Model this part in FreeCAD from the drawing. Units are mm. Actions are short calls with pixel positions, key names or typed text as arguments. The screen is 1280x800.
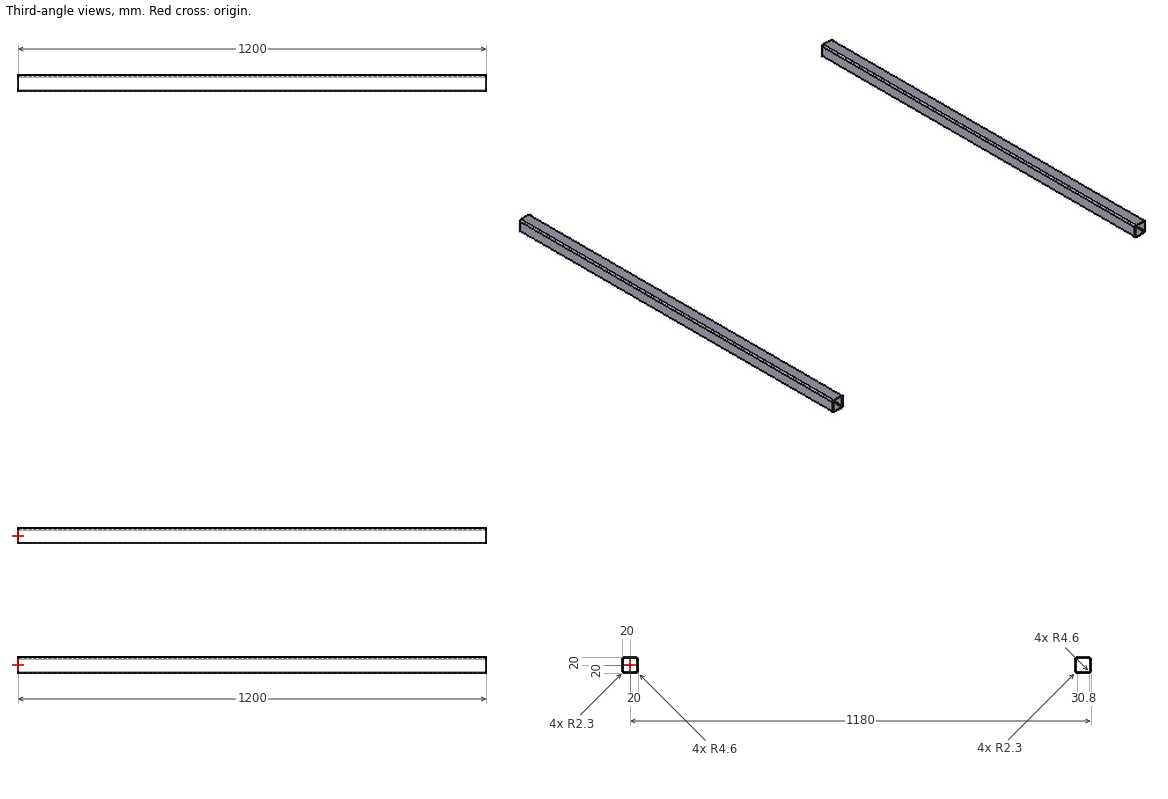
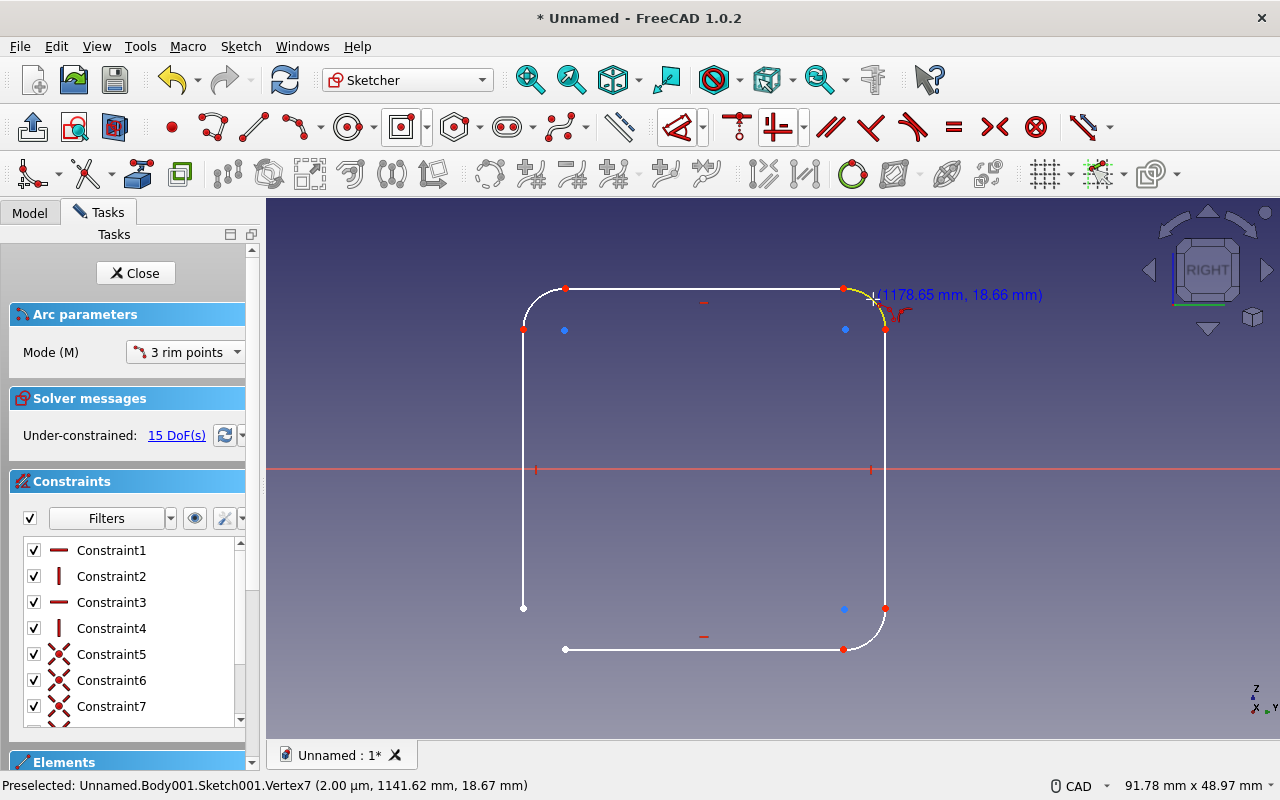
click(523, 609)
click(565, 650)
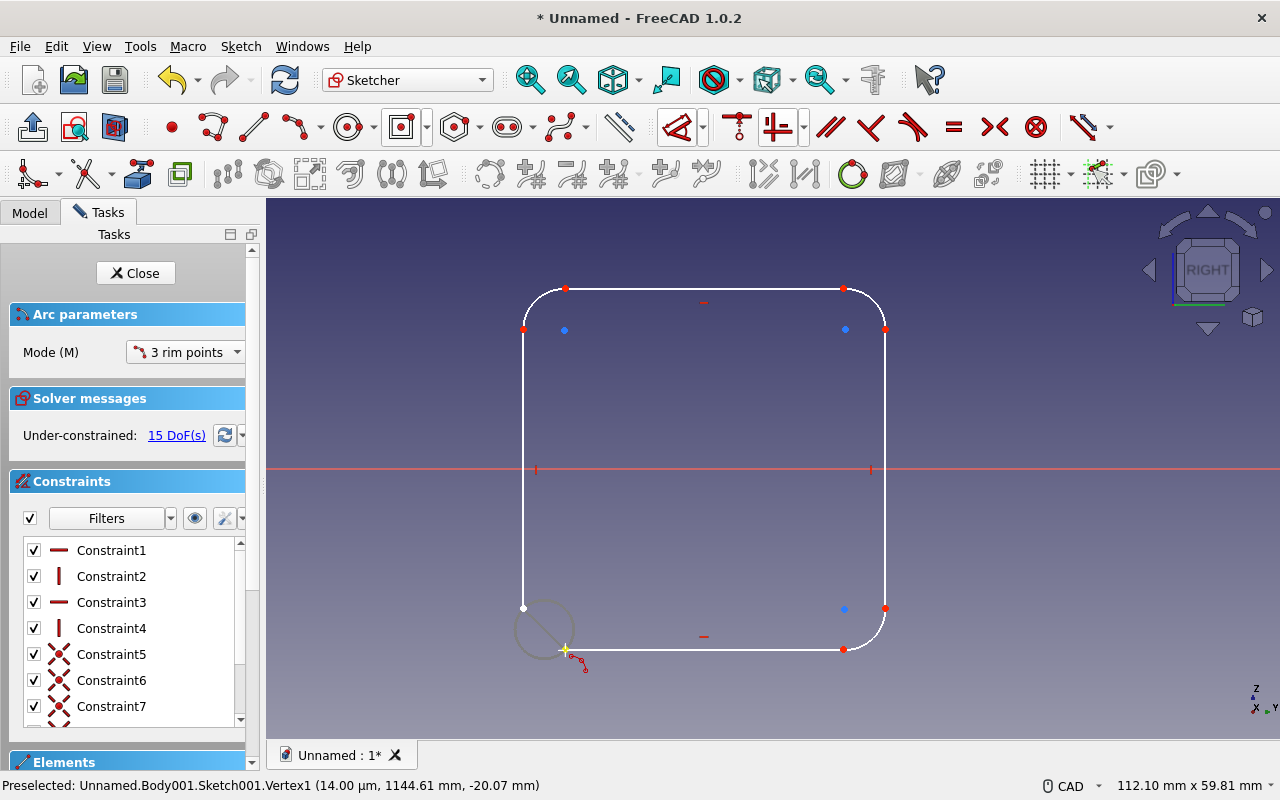
scroll(536, 637, up, 2)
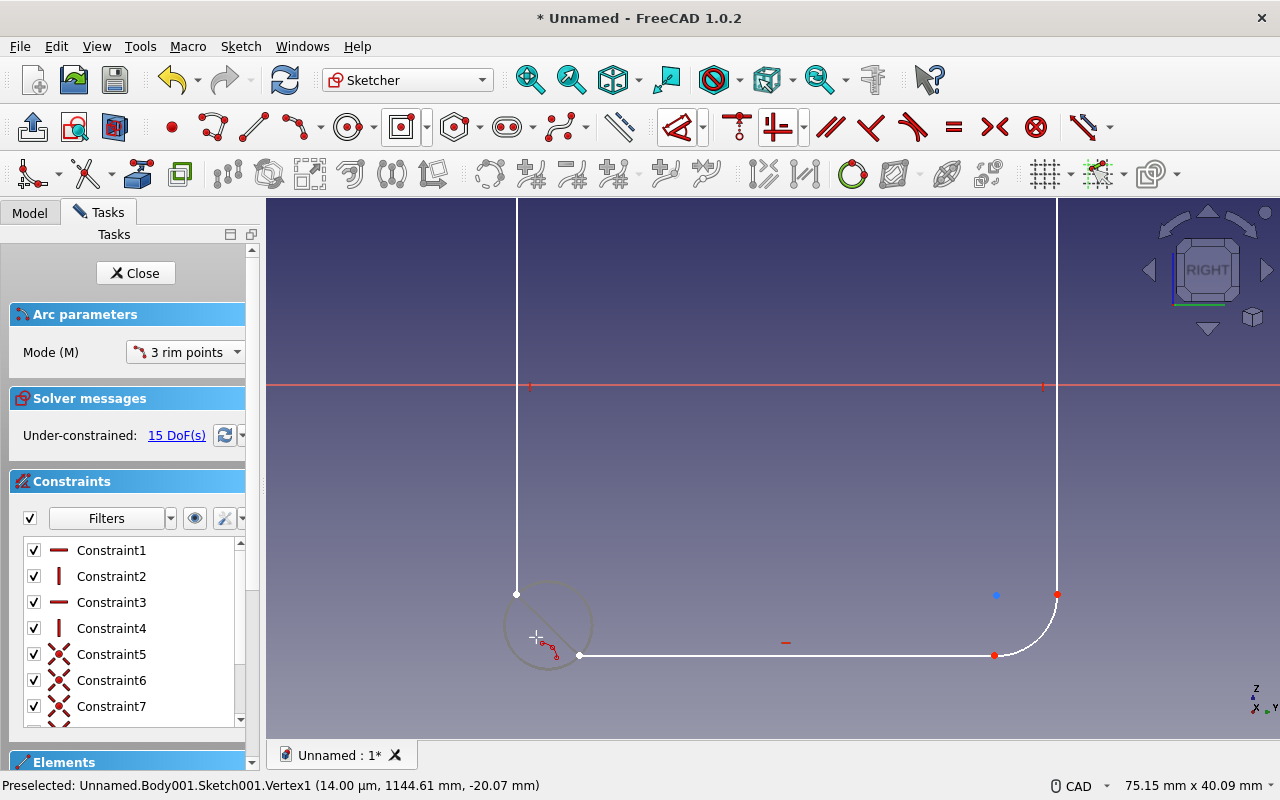
click(536, 637)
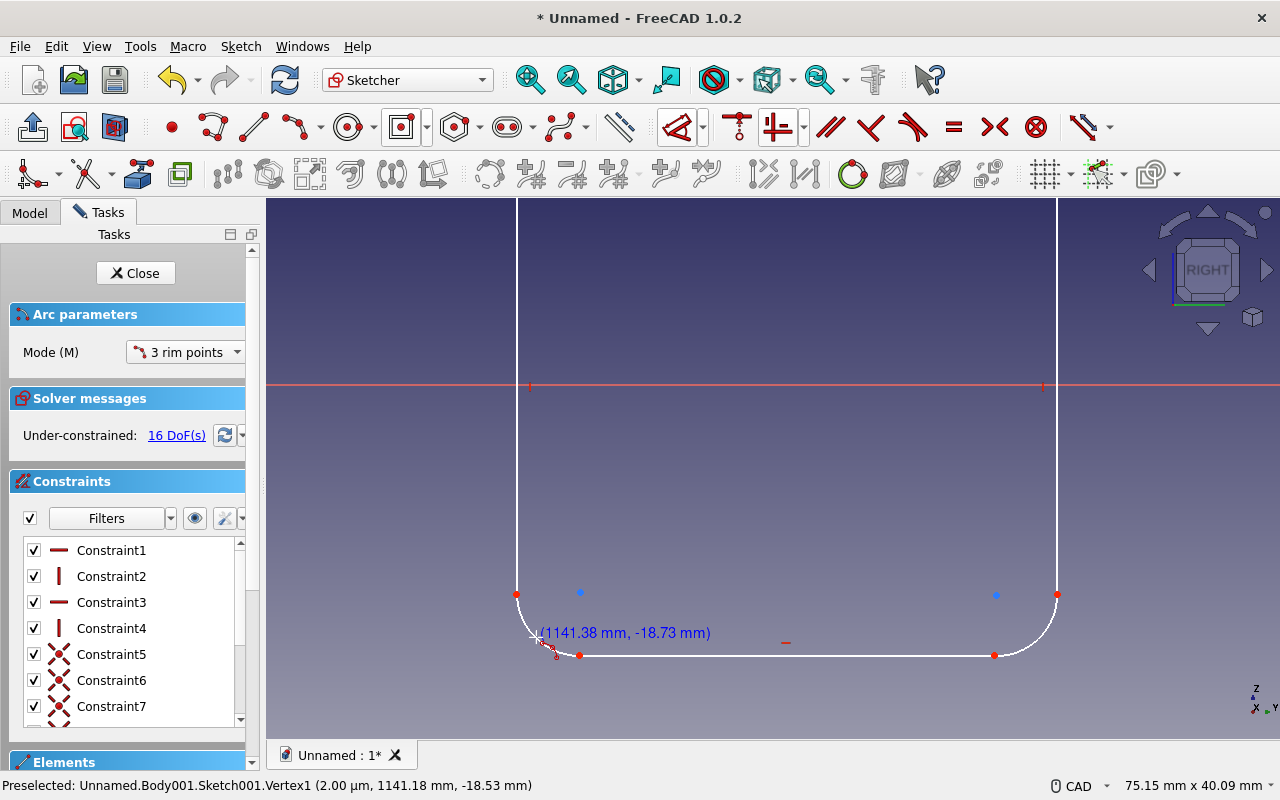
key(g)
key(l)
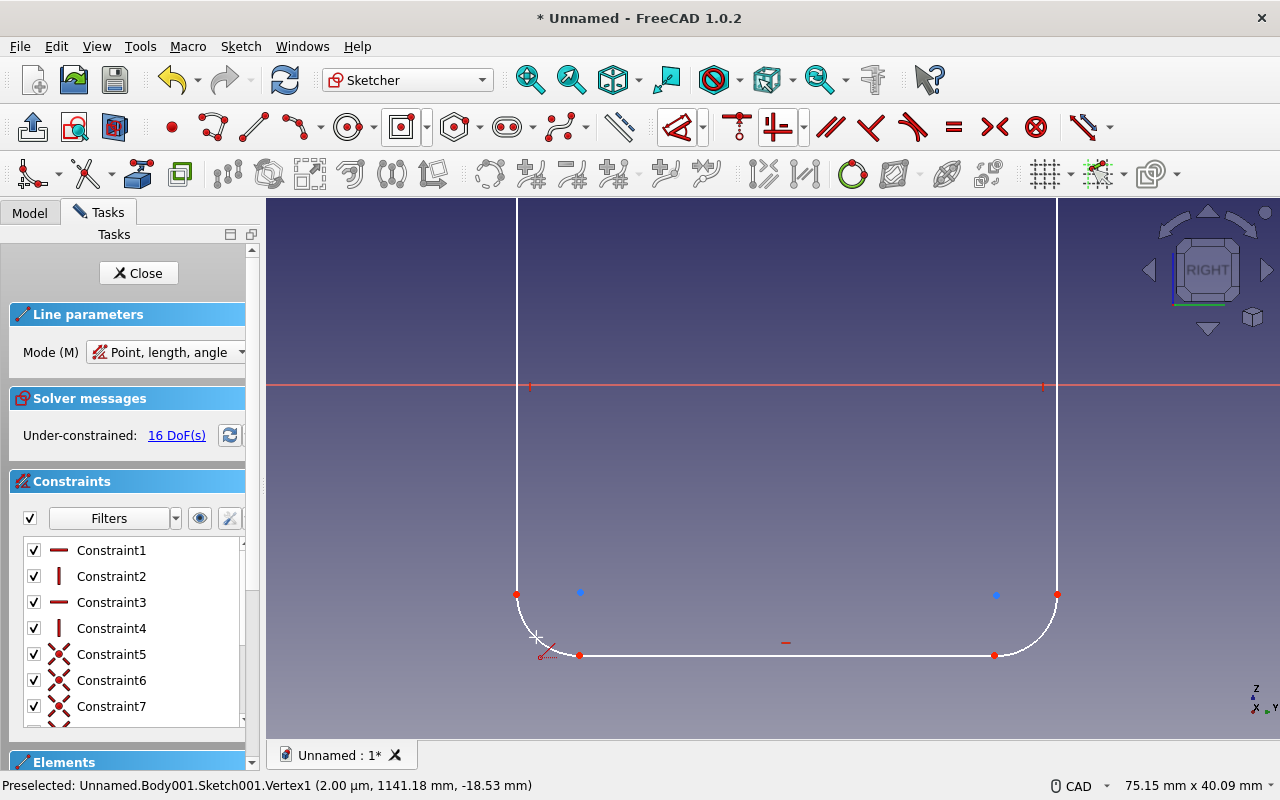
click(995, 624)
click(579, 624)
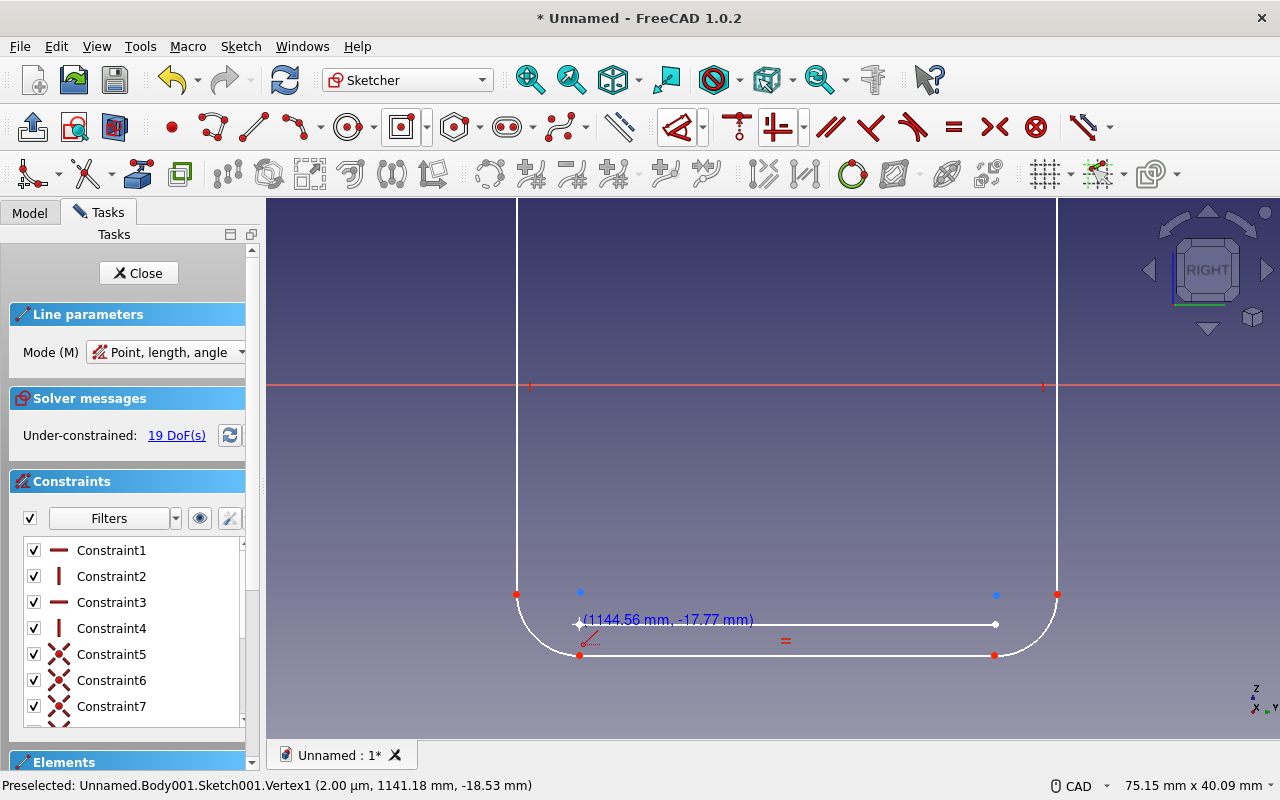
click(548, 593)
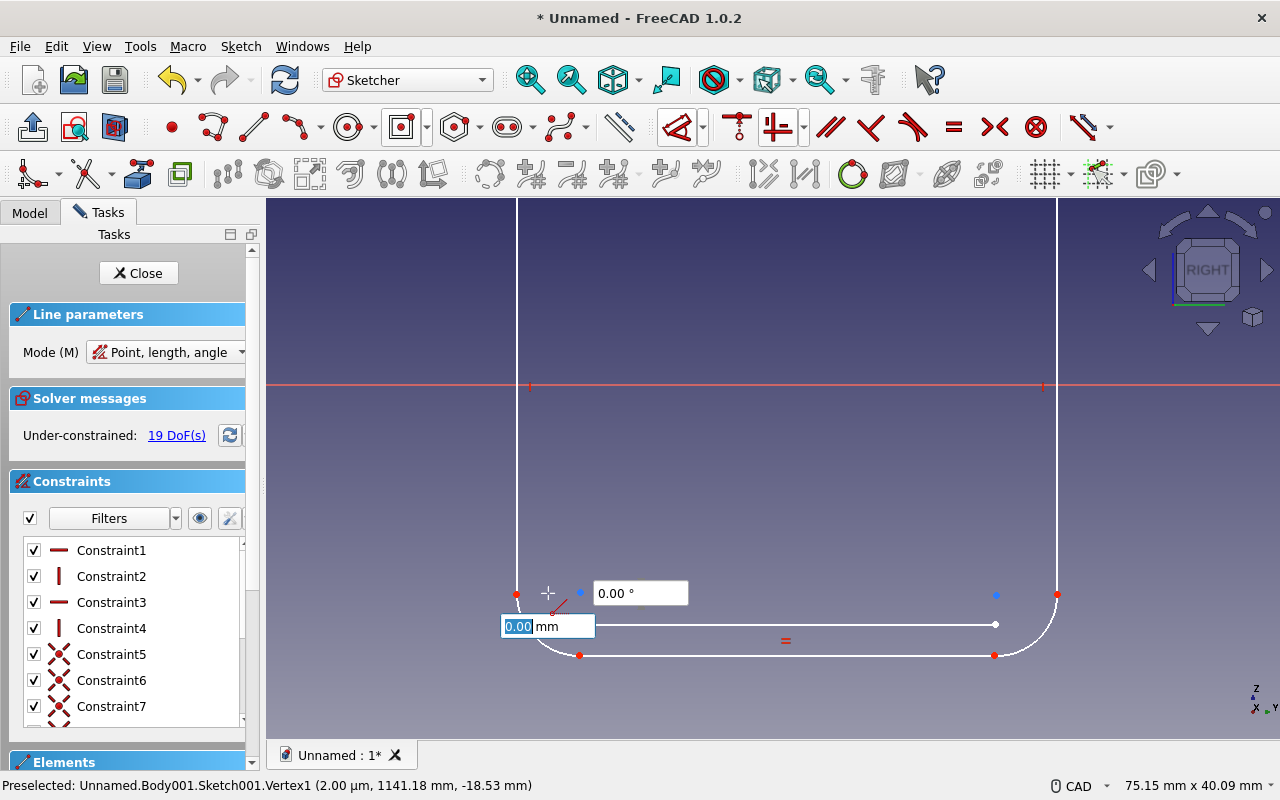
scroll(536, 638, down, 2)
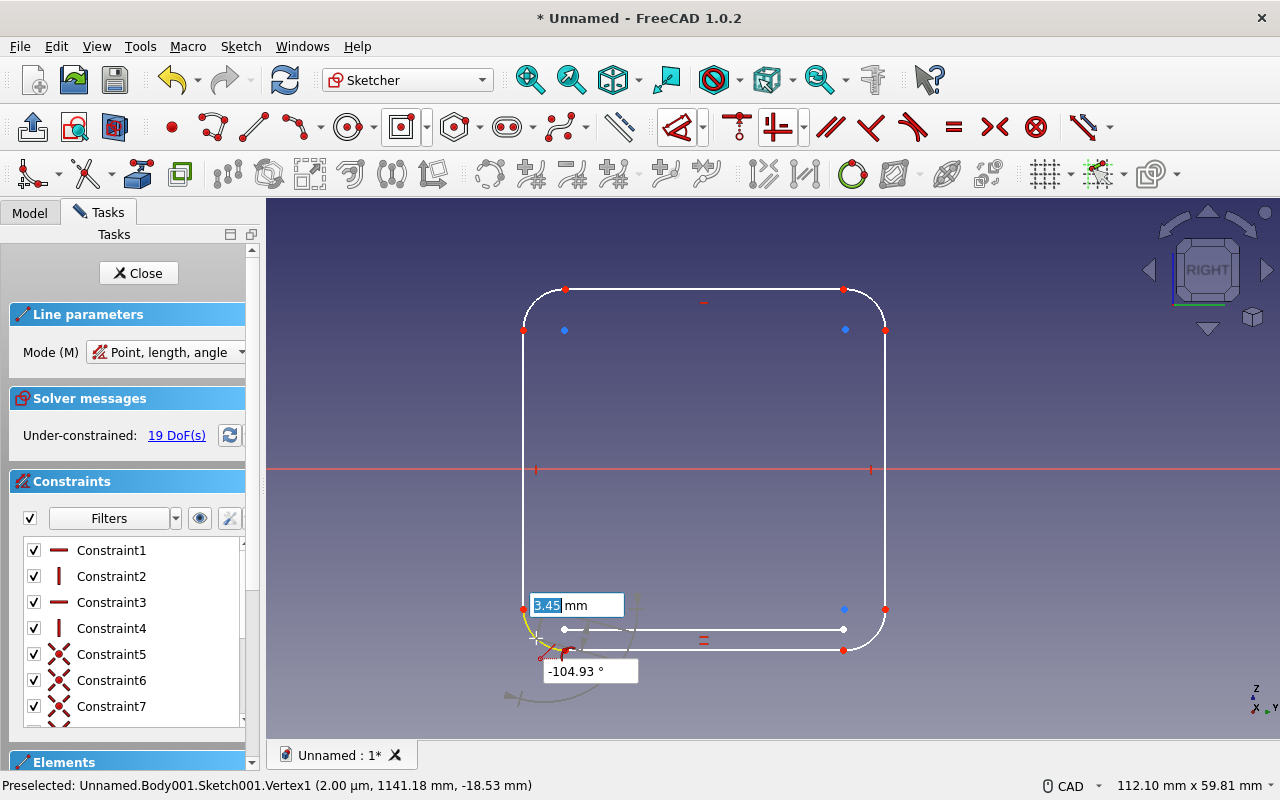
click(544, 330)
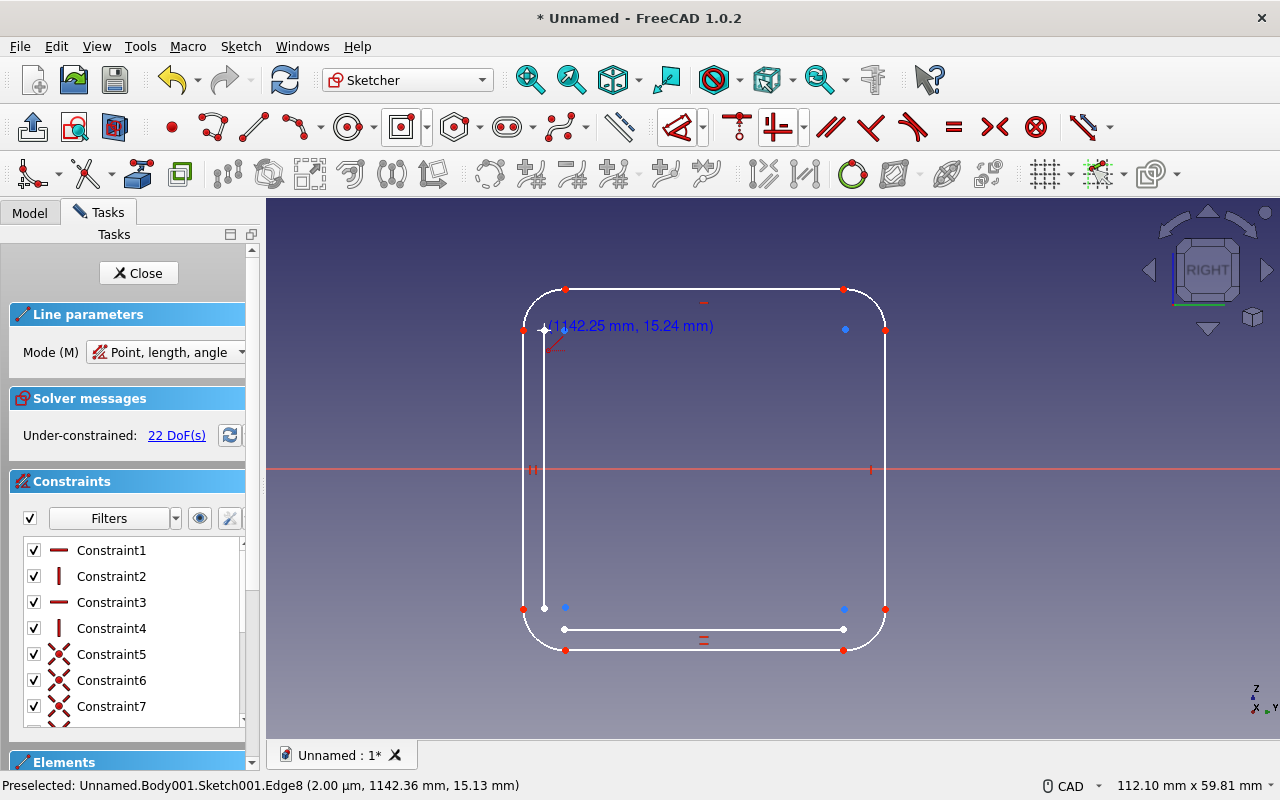
click(565, 309)
click(844, 309)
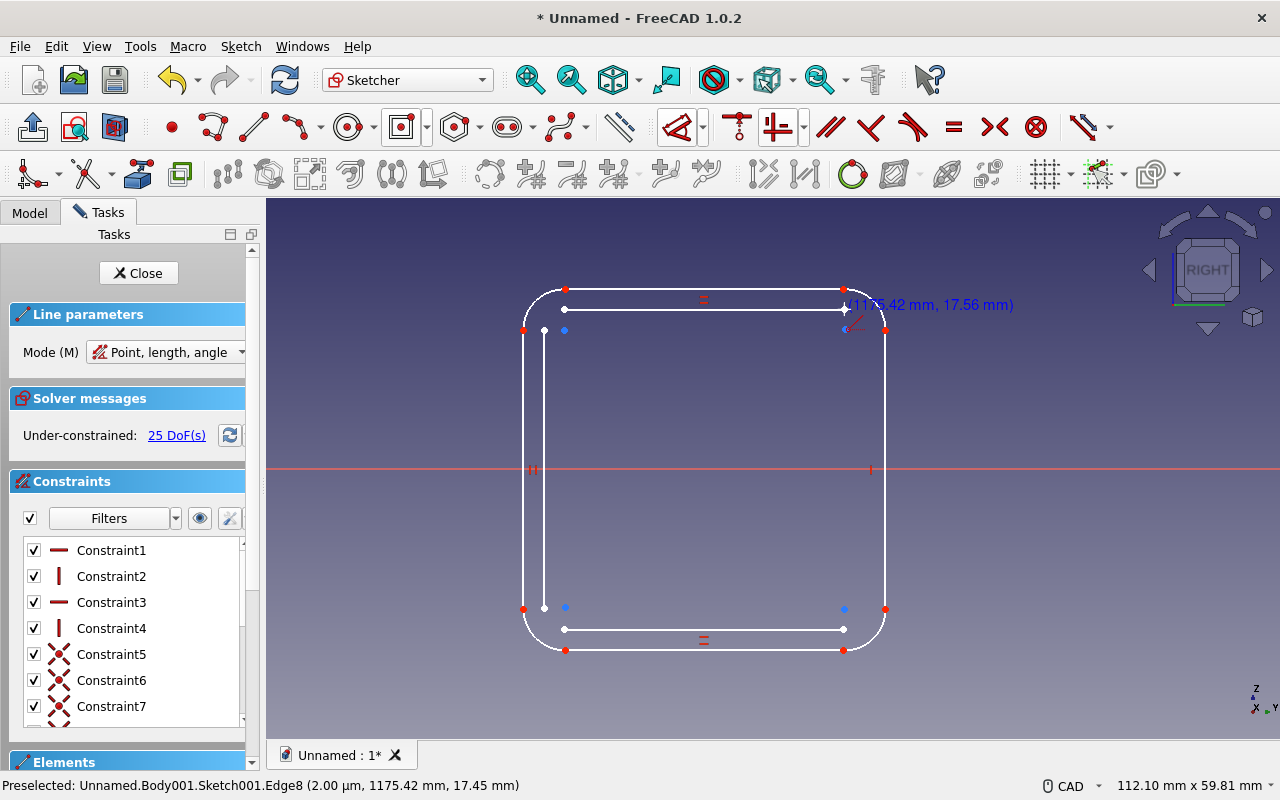
click(865, 330)
click(865, 608)